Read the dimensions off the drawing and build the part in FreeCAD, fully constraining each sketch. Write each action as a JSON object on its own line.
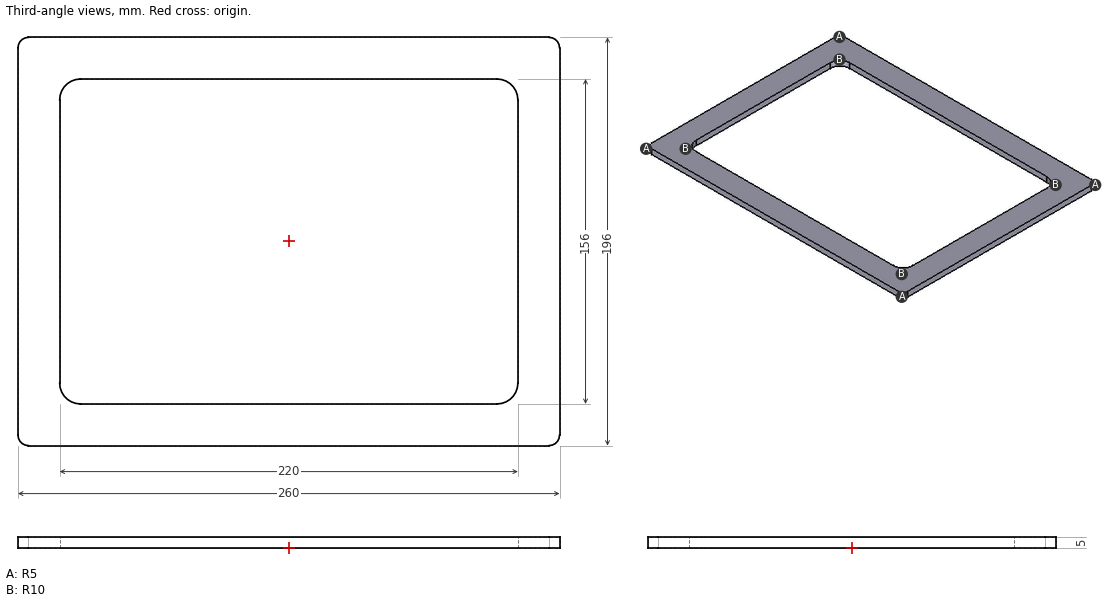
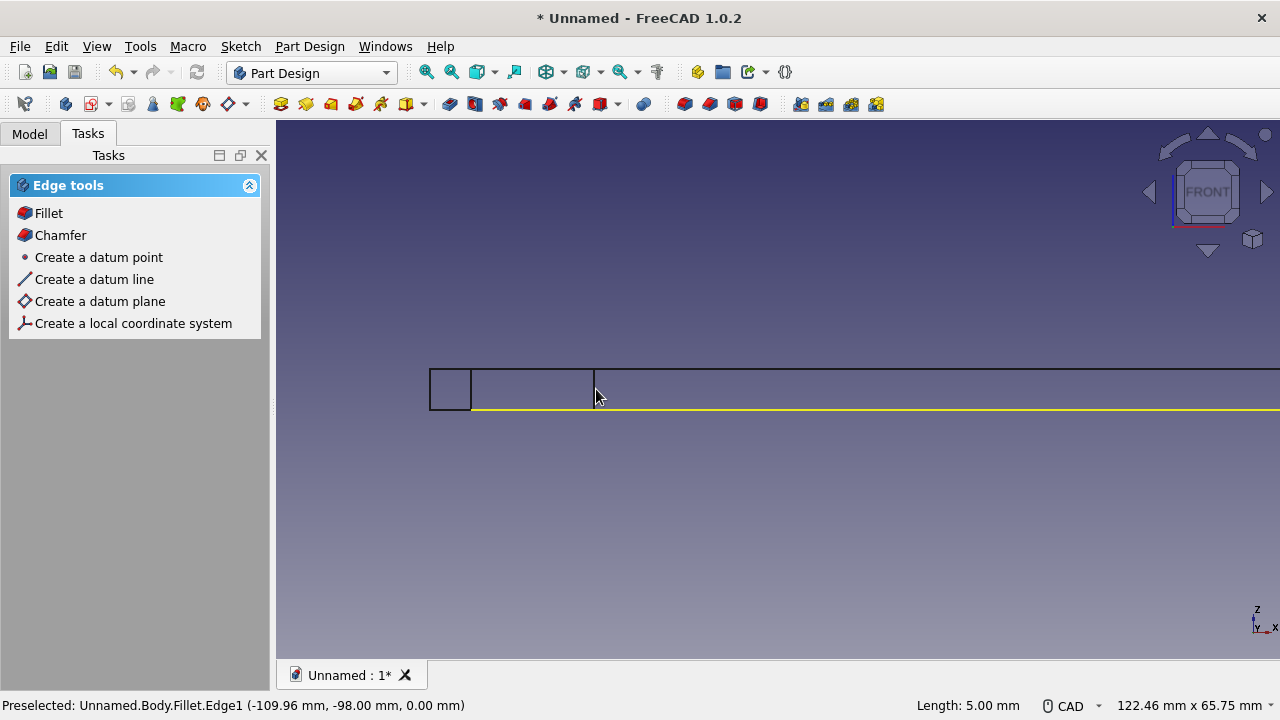
{"action": "left_click", "coordinate": [594, 389], "text": "ctrl"}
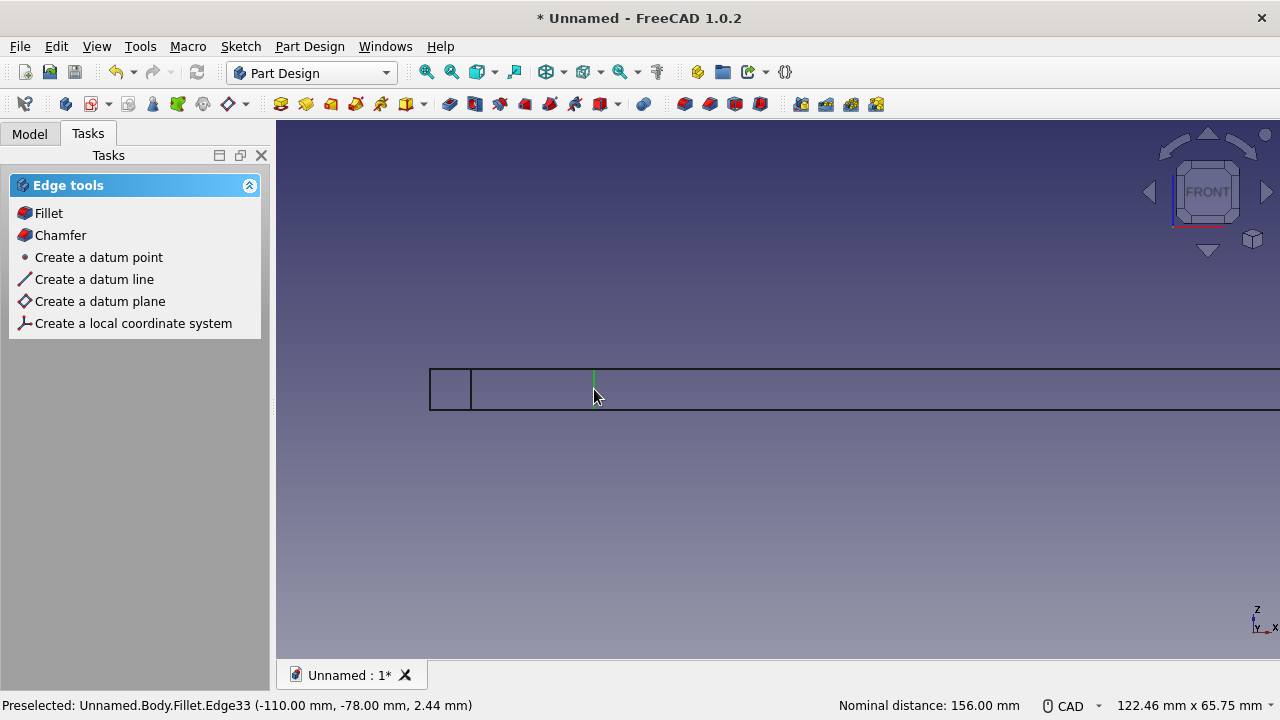
{"action": "left_click", "coordinate": [427, 72]}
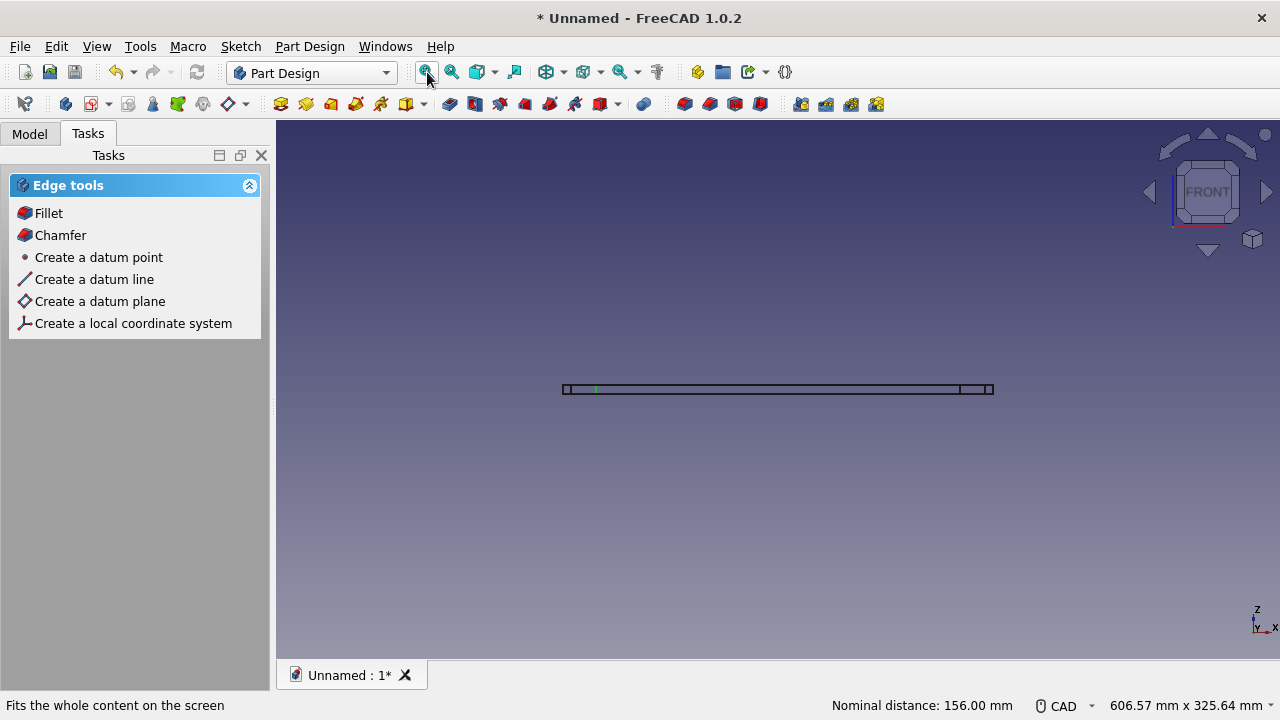
{"action": "key", "text": "3"}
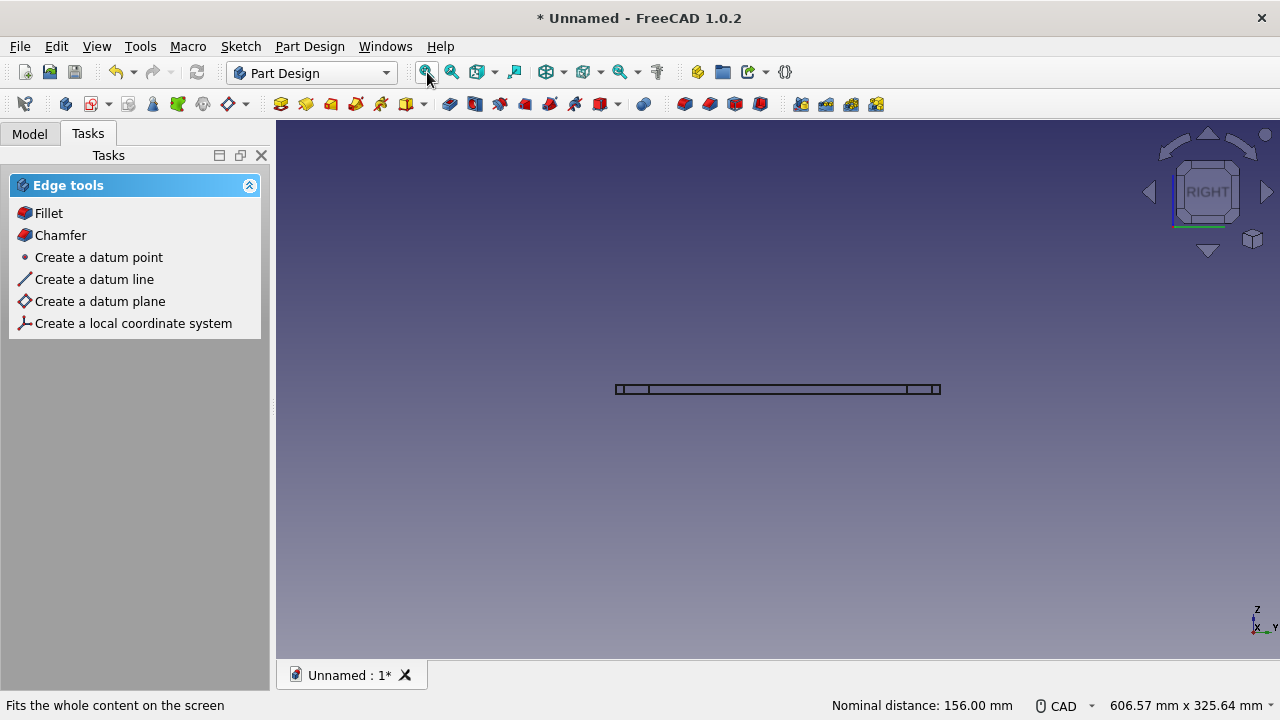
{"action": "left_click", "coordinate": [427, 72]}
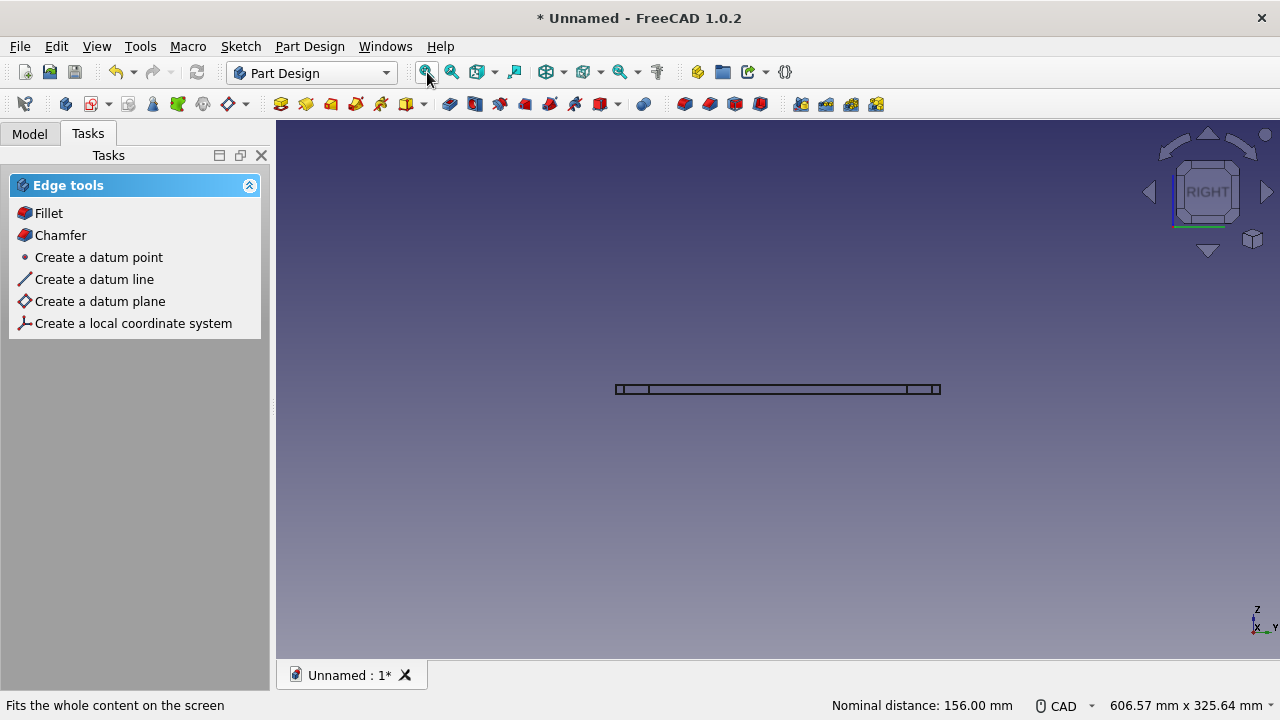
{"action": "scroll", "coordinate": [649, 388], "scroll_direction": "up", "scroll_amount": 8}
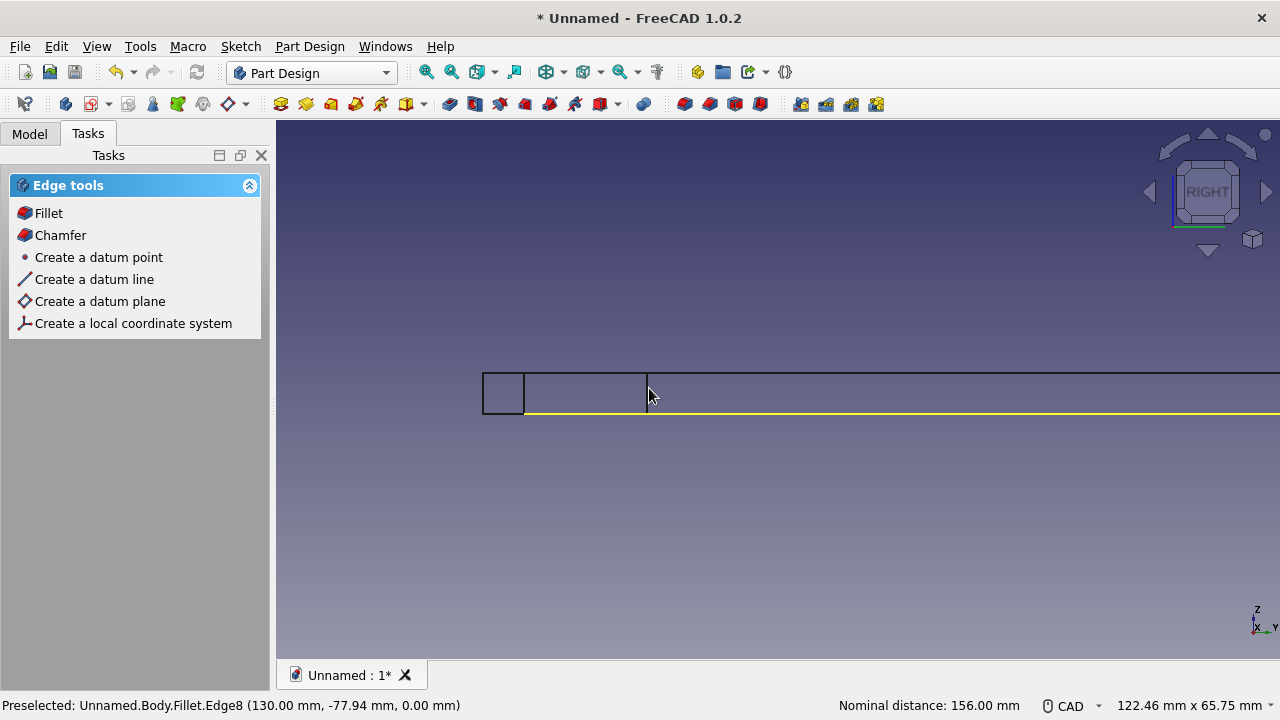
{"action": "left_click", "coordinate": [647, 392], "text": "ctrl"}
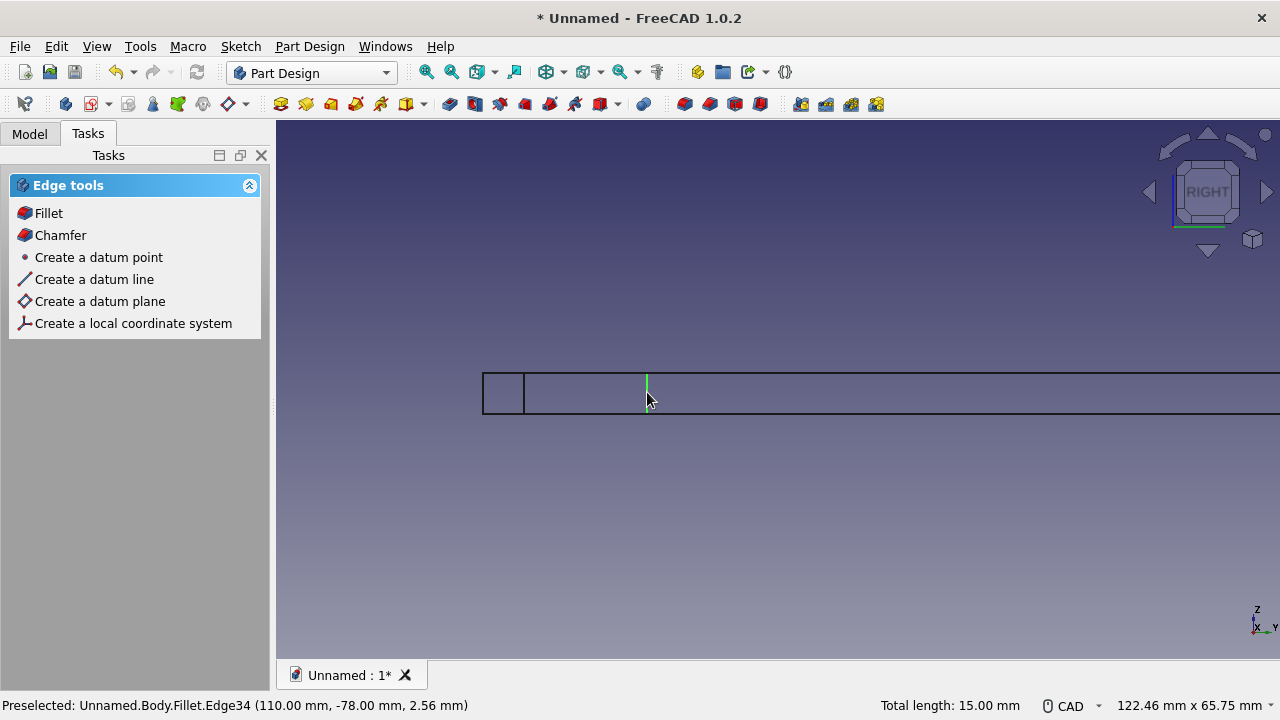
{"action": "left_click", "coordinate": [427, 72]}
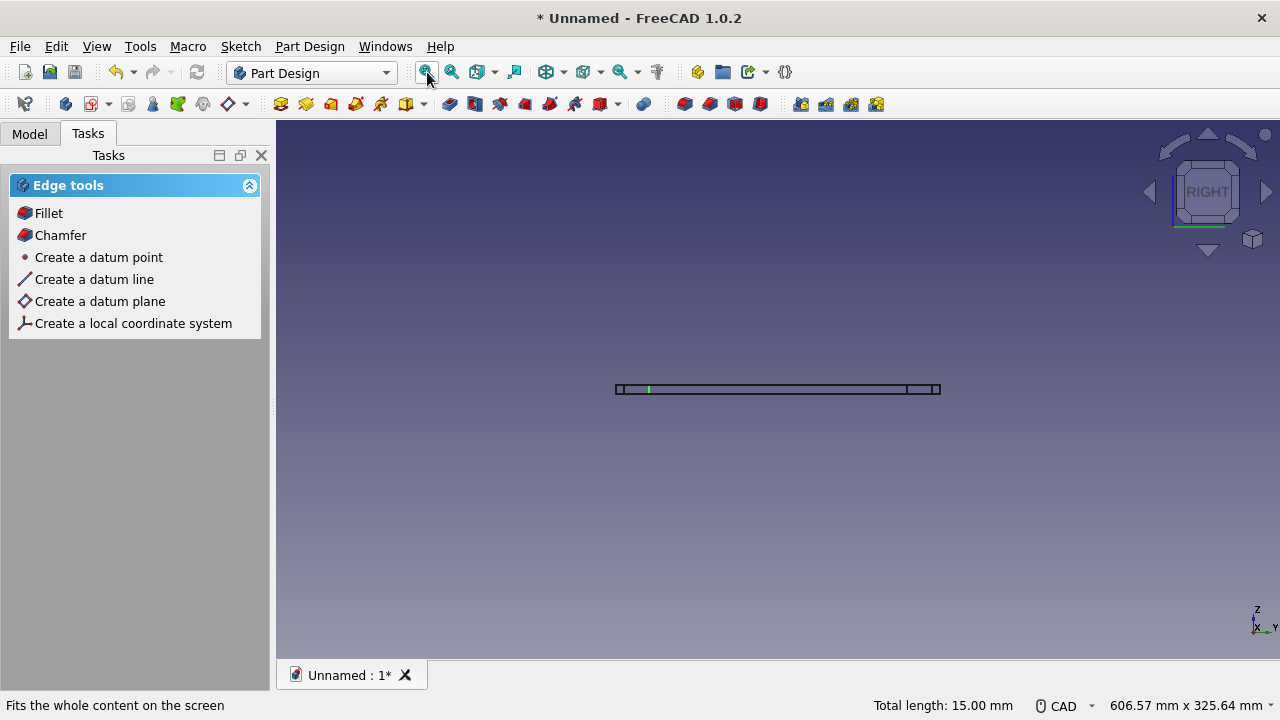
{"action": "key", "text": "5"}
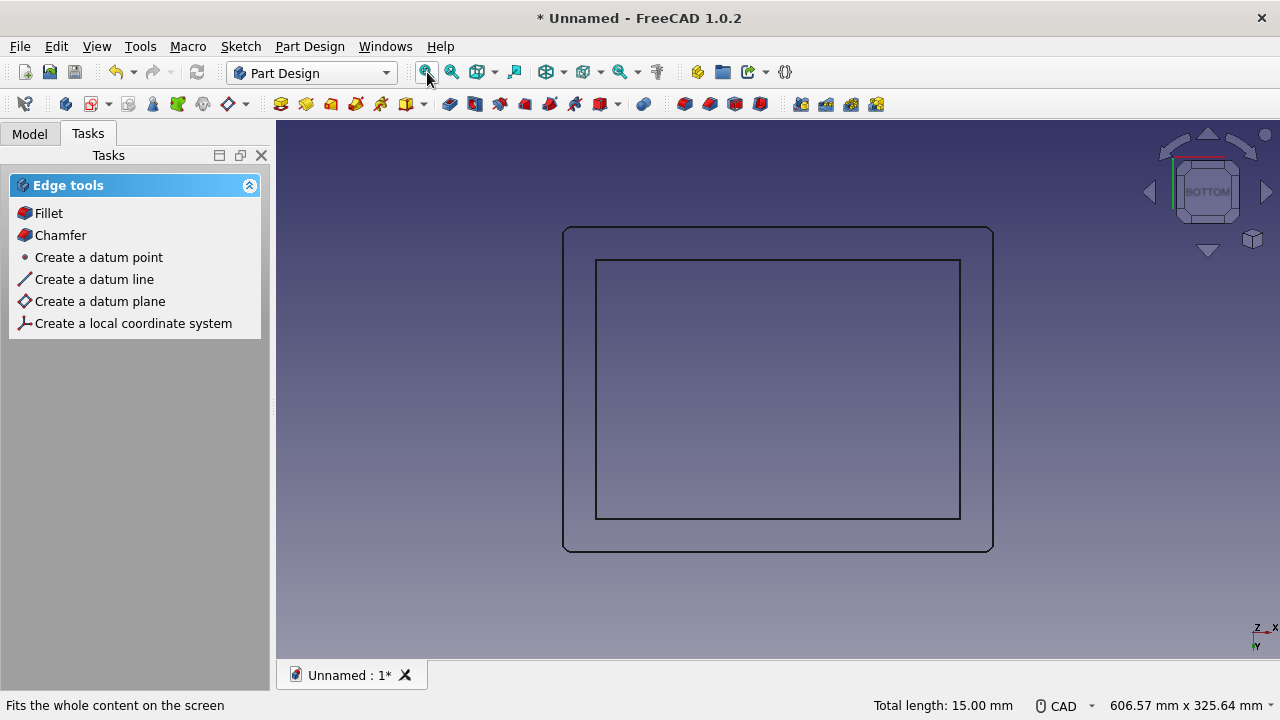
{"action": "scroll", "coordinate": [960, 518], "scroll_direction": "up", "scroll_amount": 8}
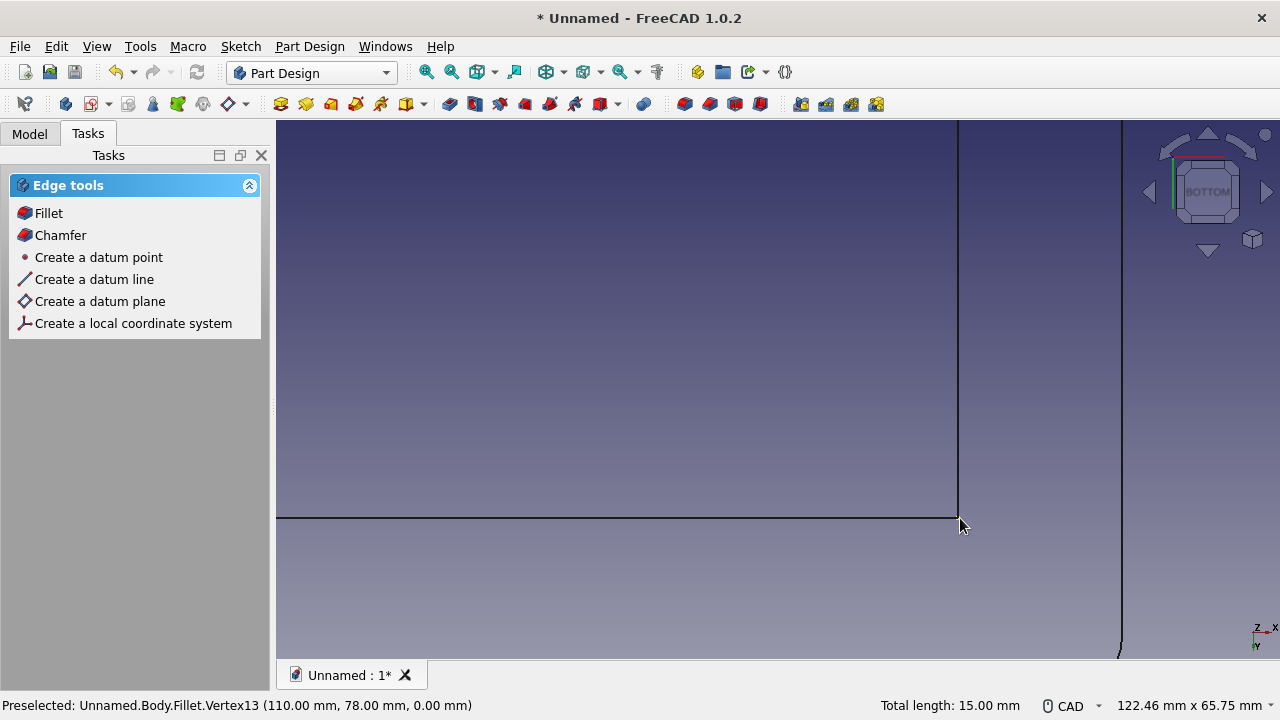
{"action": "key", "text": "v f"}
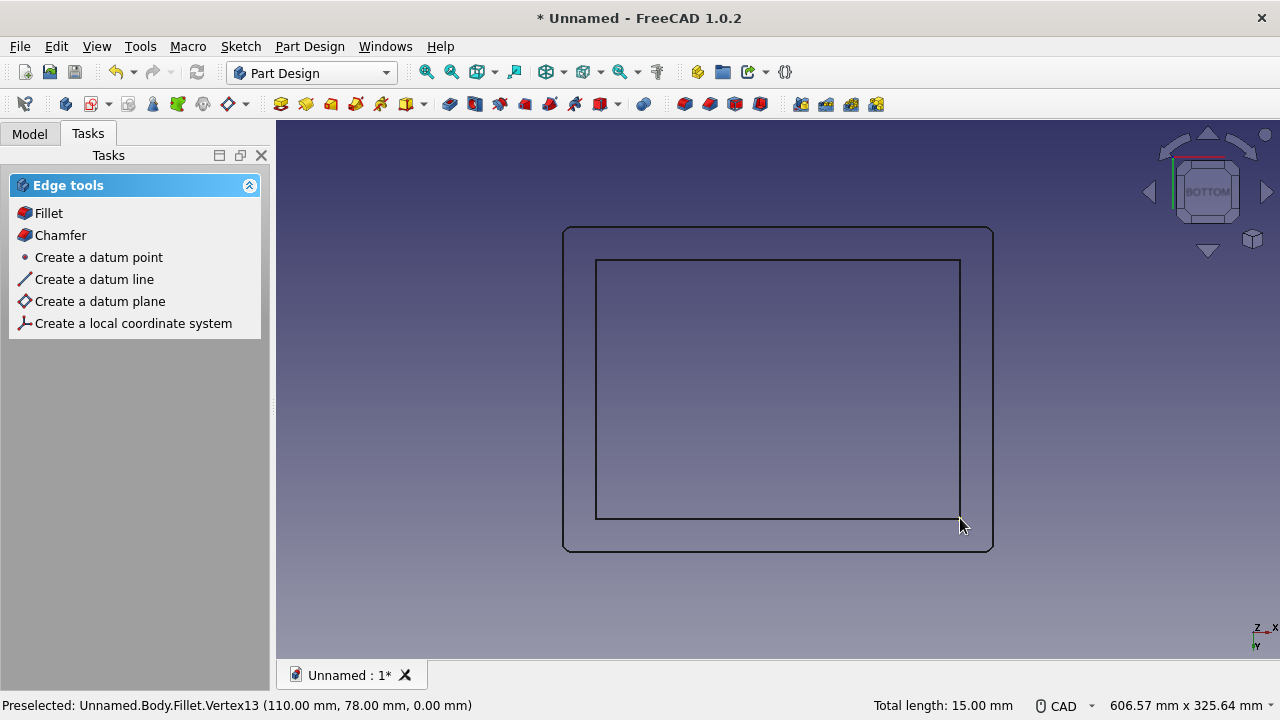
{"action": "key", "text": "4"}